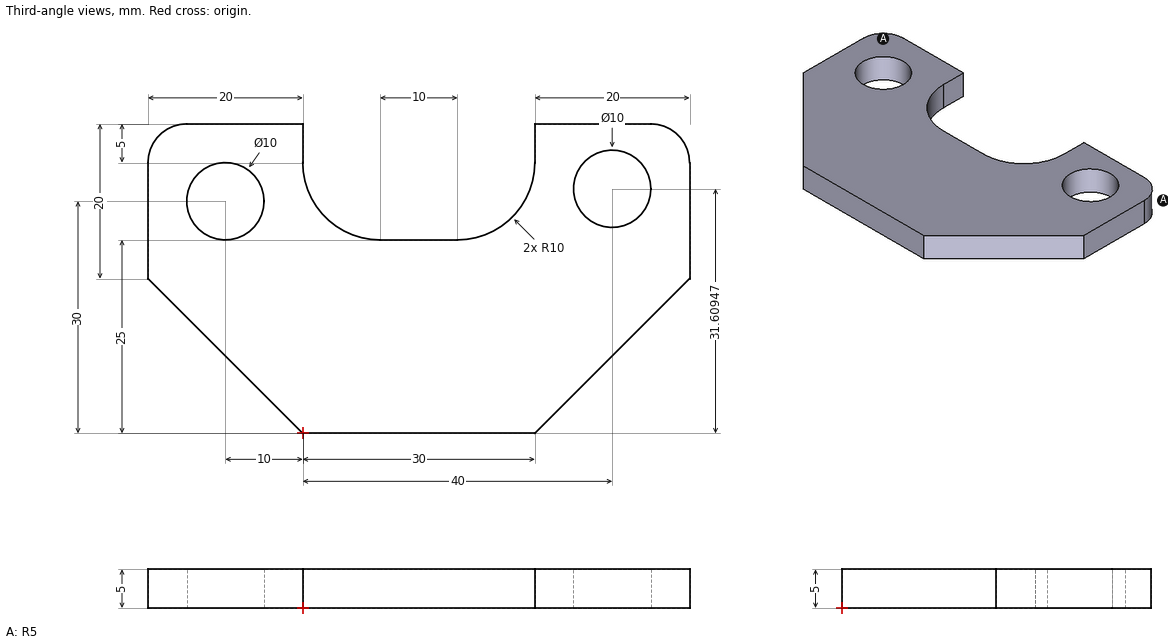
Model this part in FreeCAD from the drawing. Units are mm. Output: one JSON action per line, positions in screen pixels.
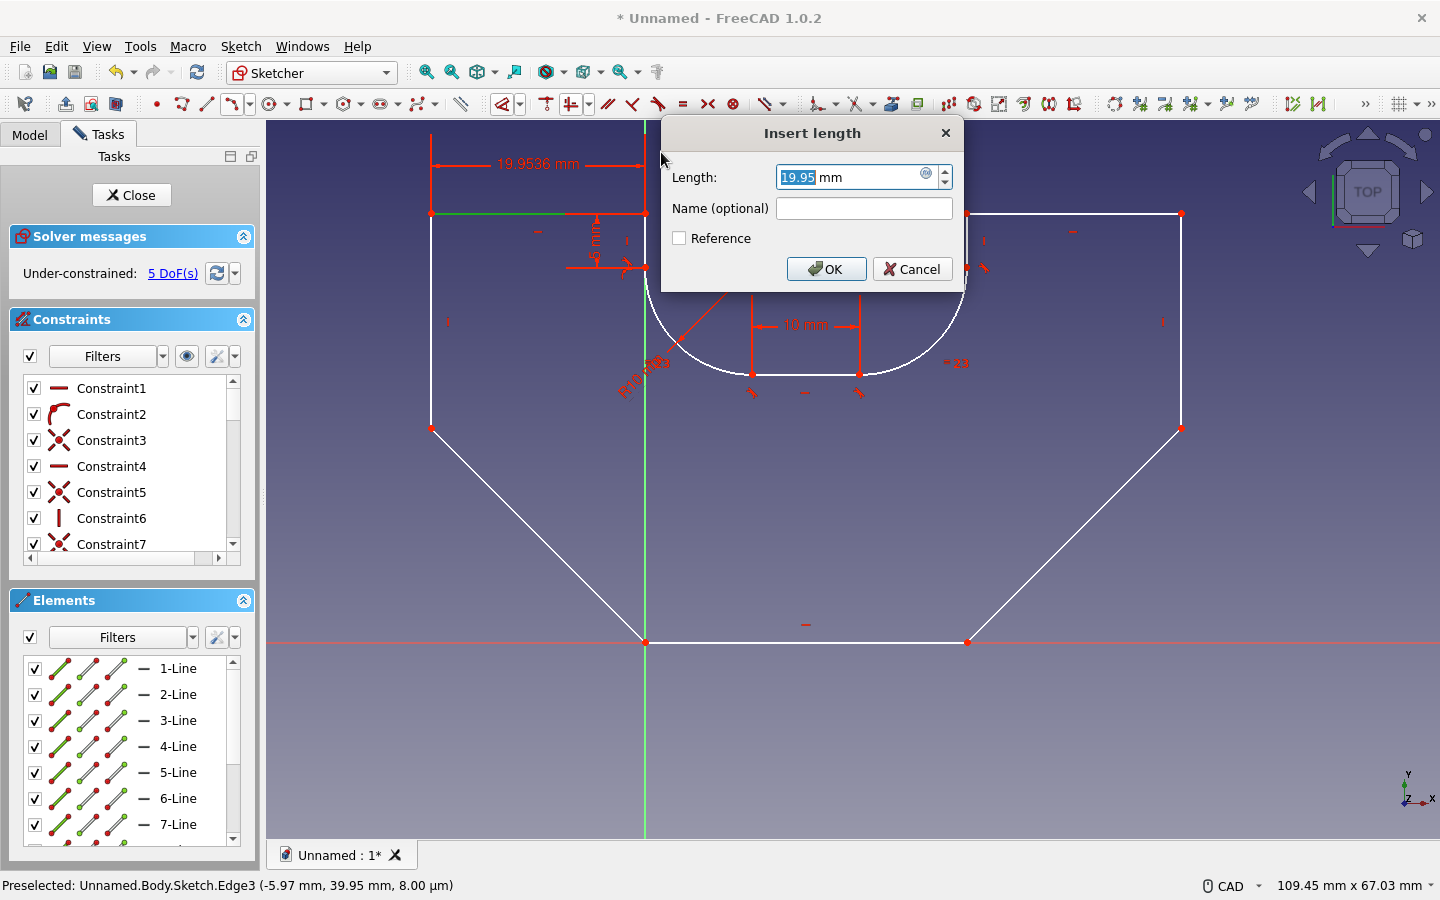
{"action": "type", "text": "20"}
{"action": "key", "text": "Return"}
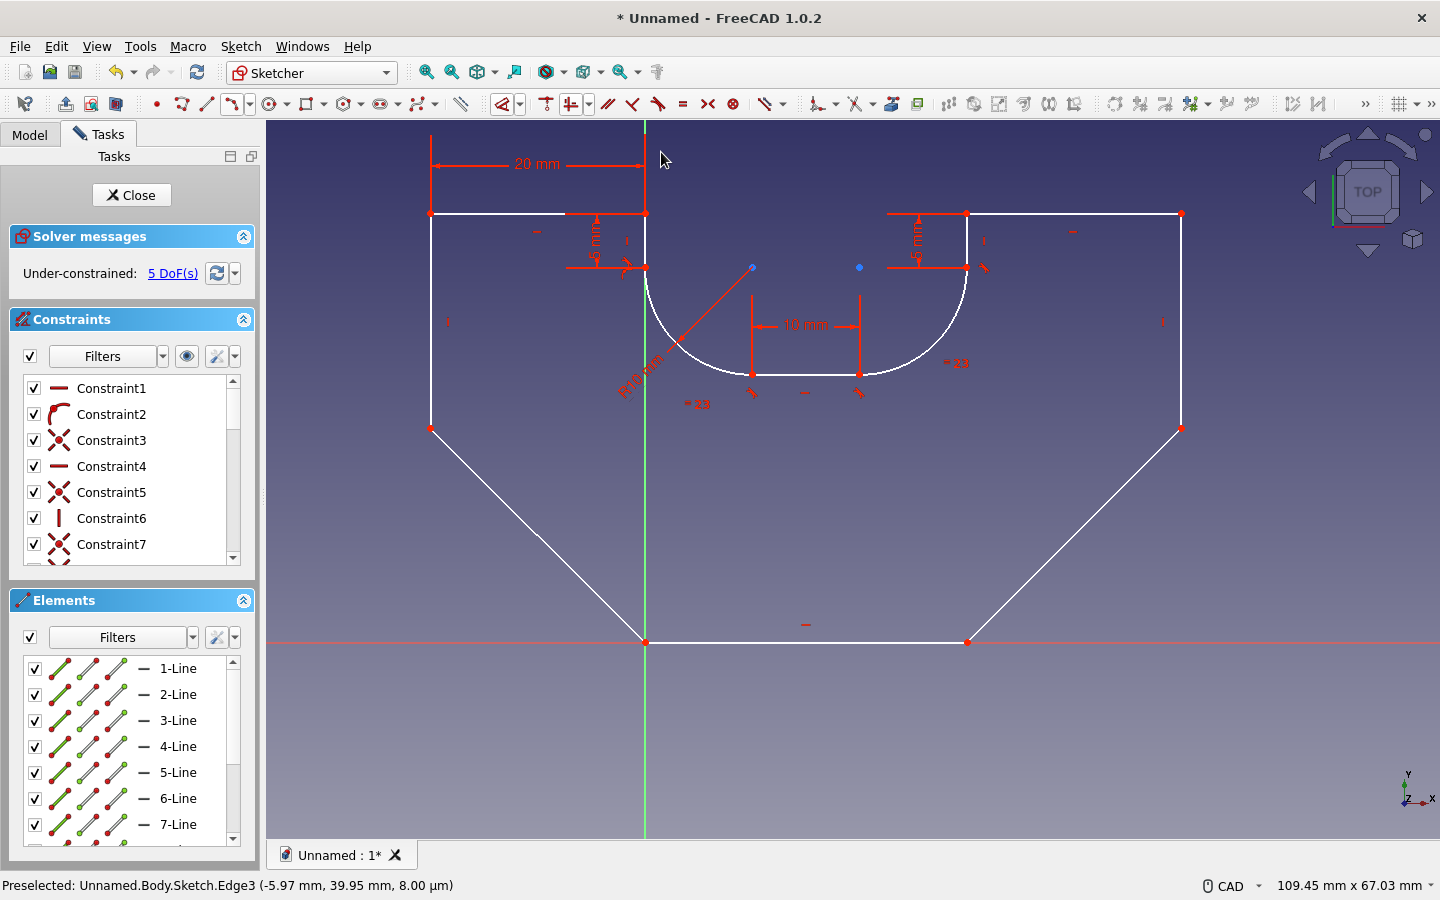
{"action": "left_click", "coordinate": [431, 278]}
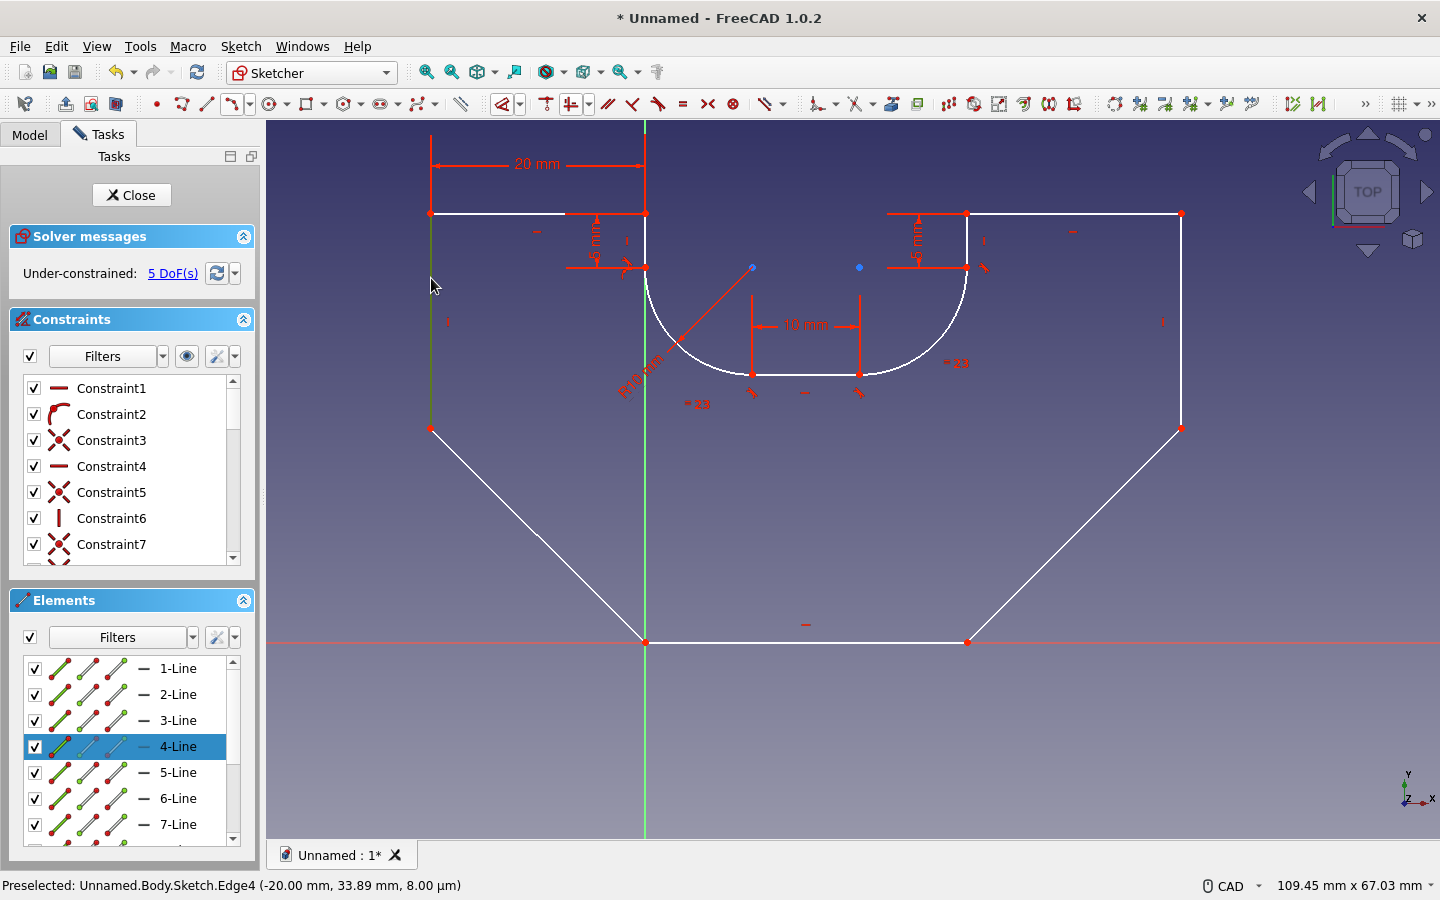
{"action": "key", "text": "i"}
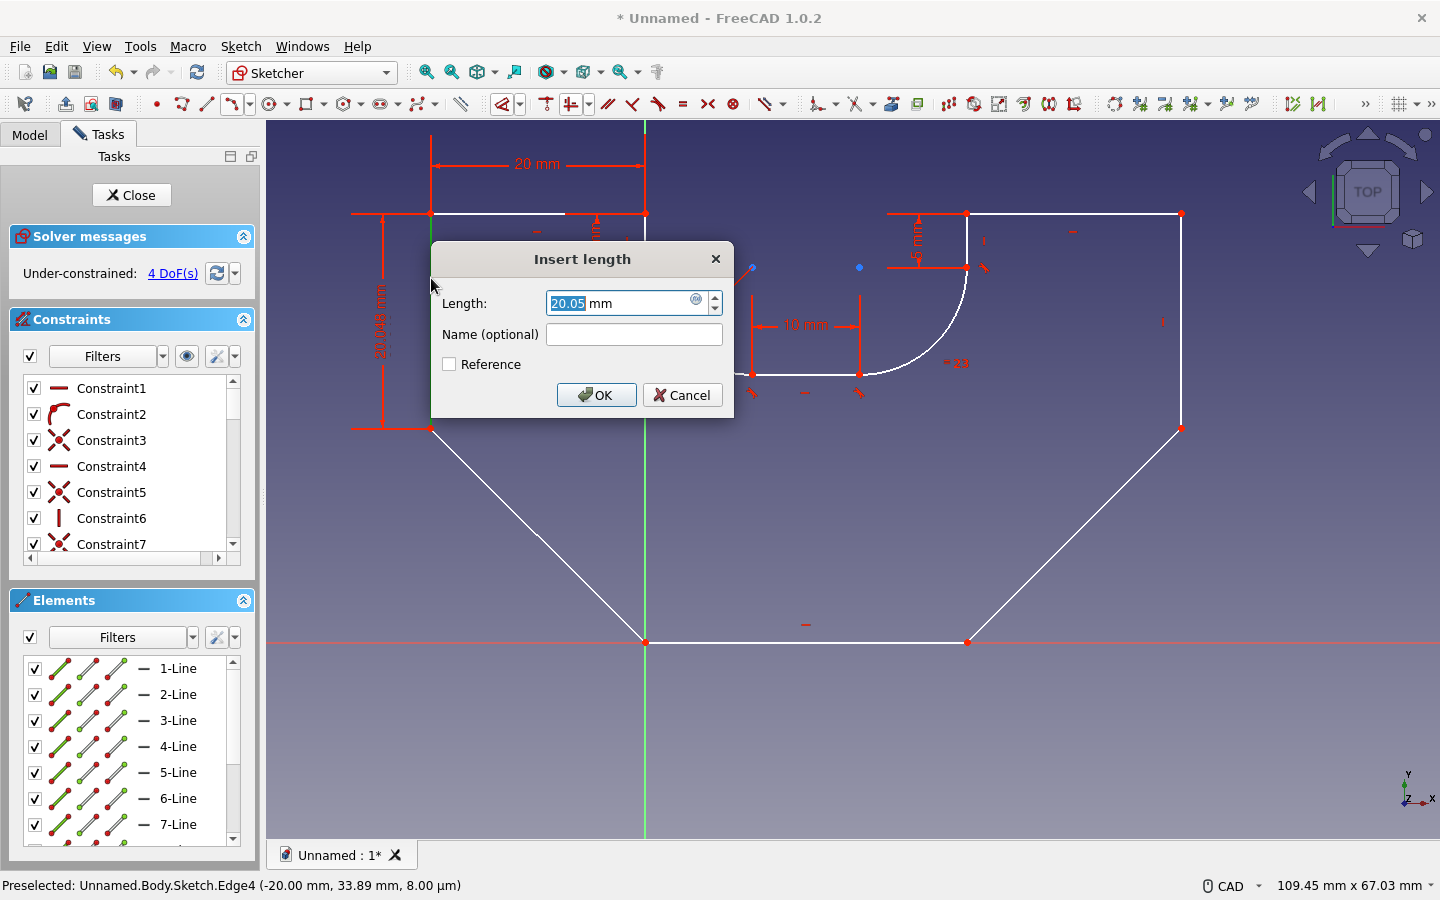
{"action": "type", "text": "20"}
{"action": "key", "text": "Return"}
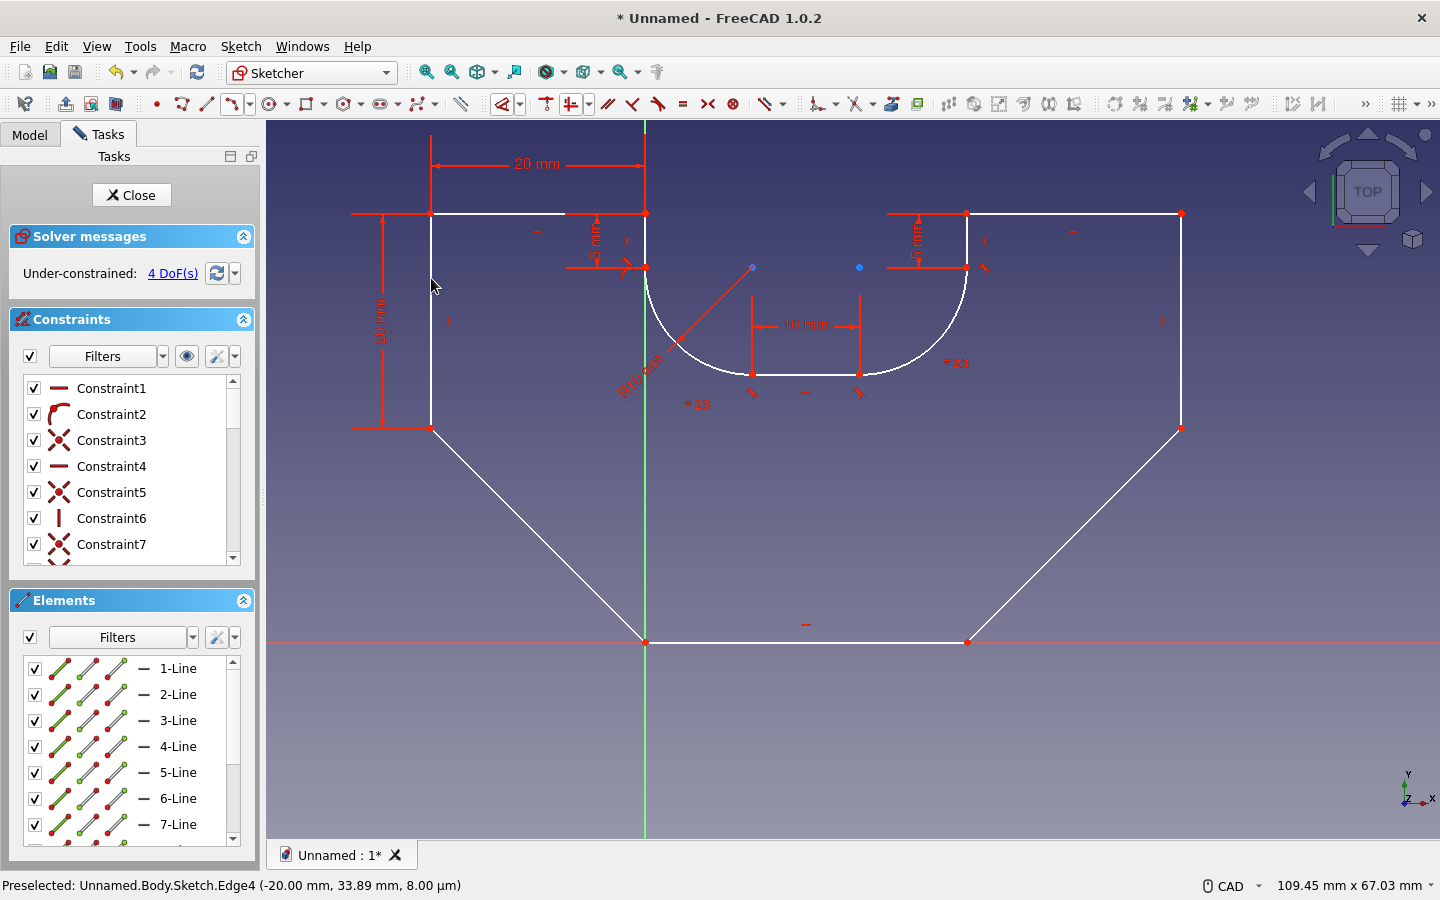
{"action": "left_click", "coordinate": [742, 643]}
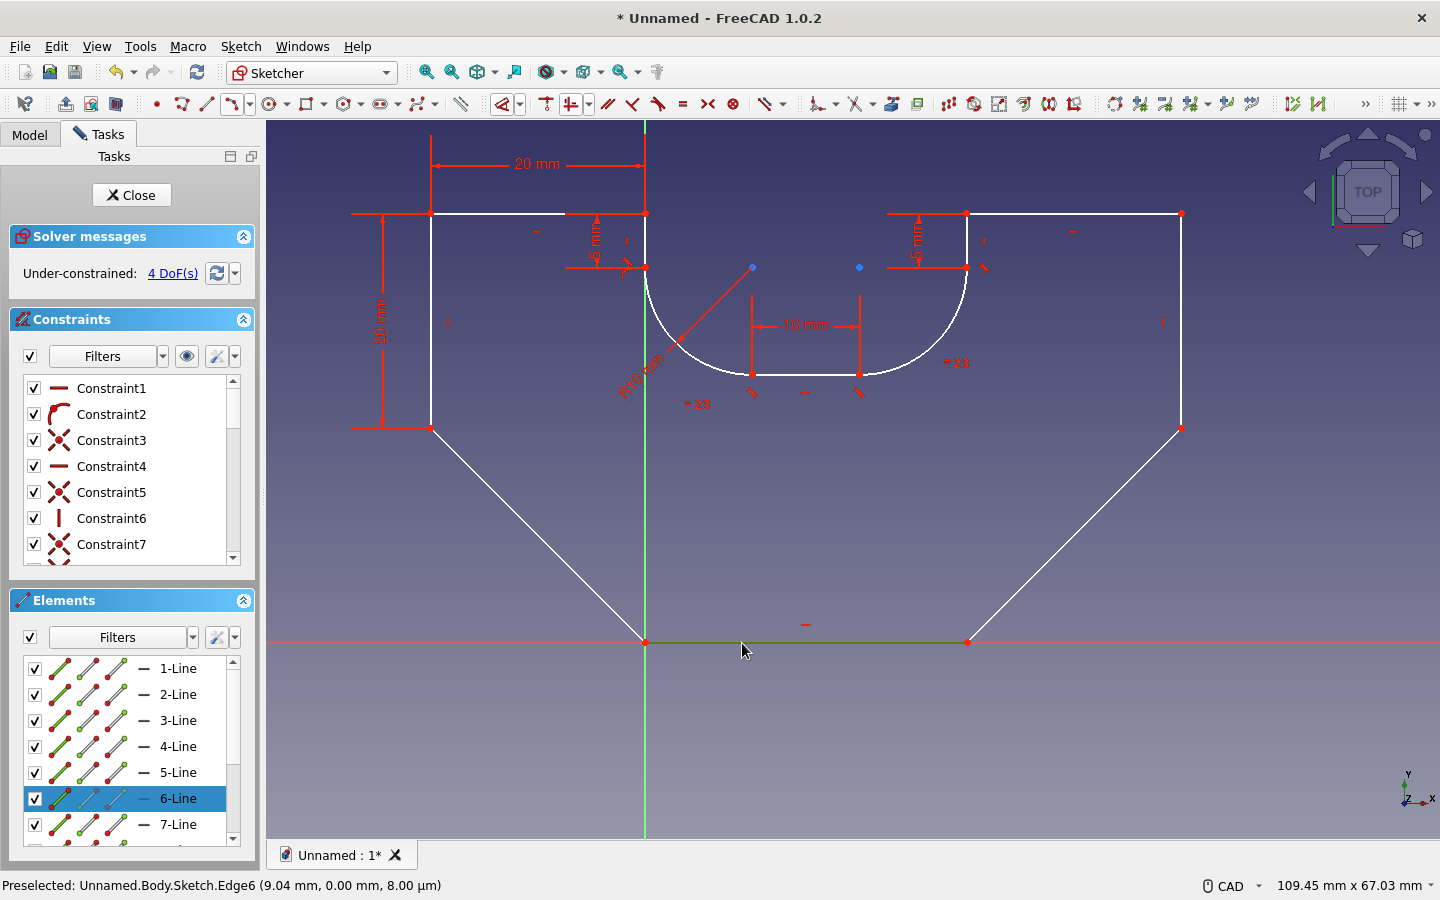
{"action": "left_click", "coordinate": [520, 104]}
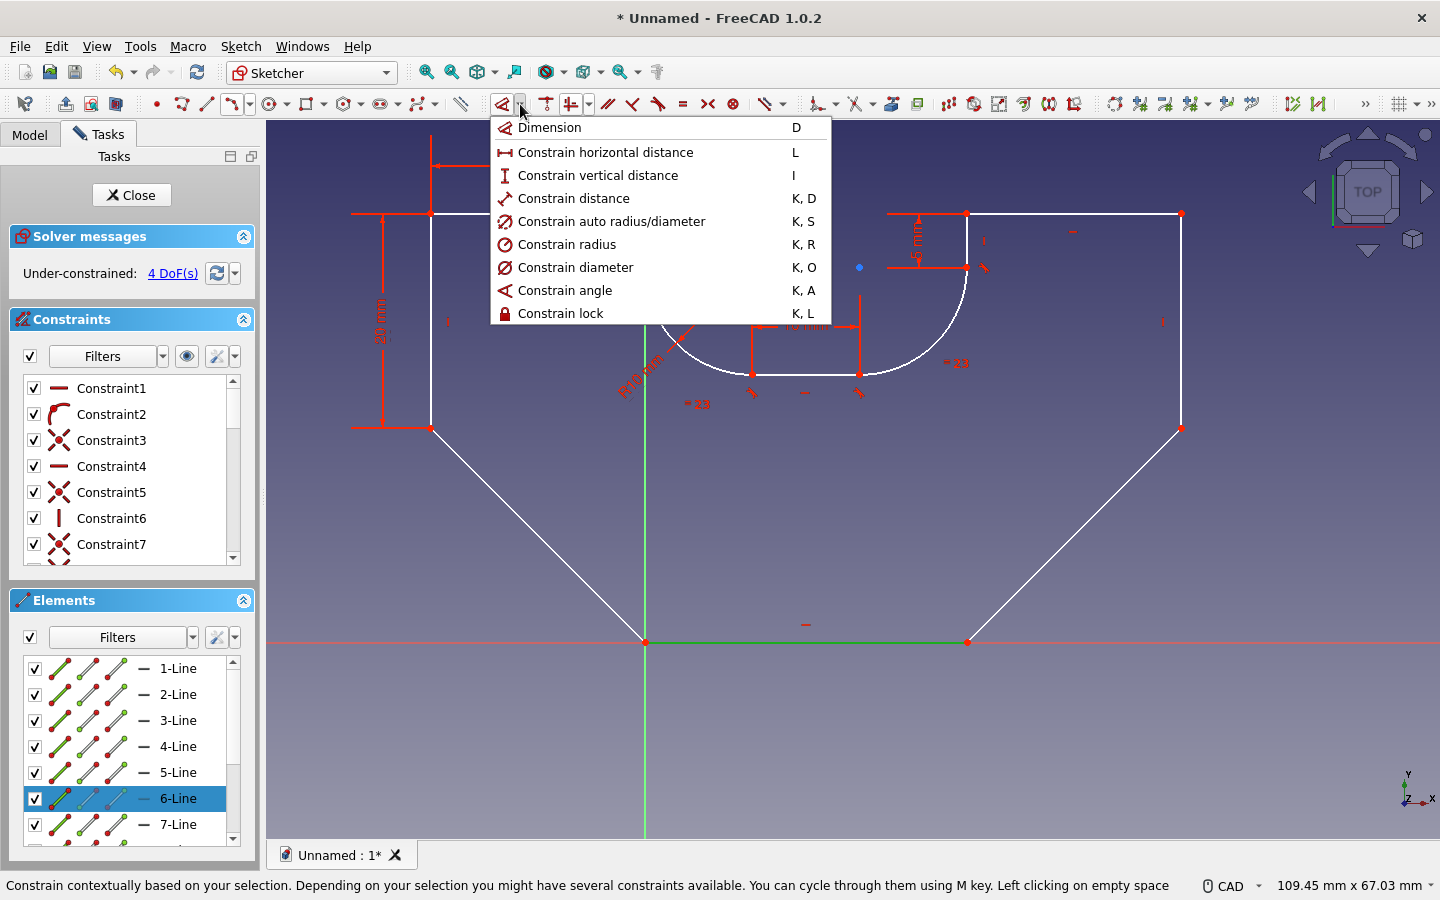
{"action": "left_click", "coordinate": [661, 152]}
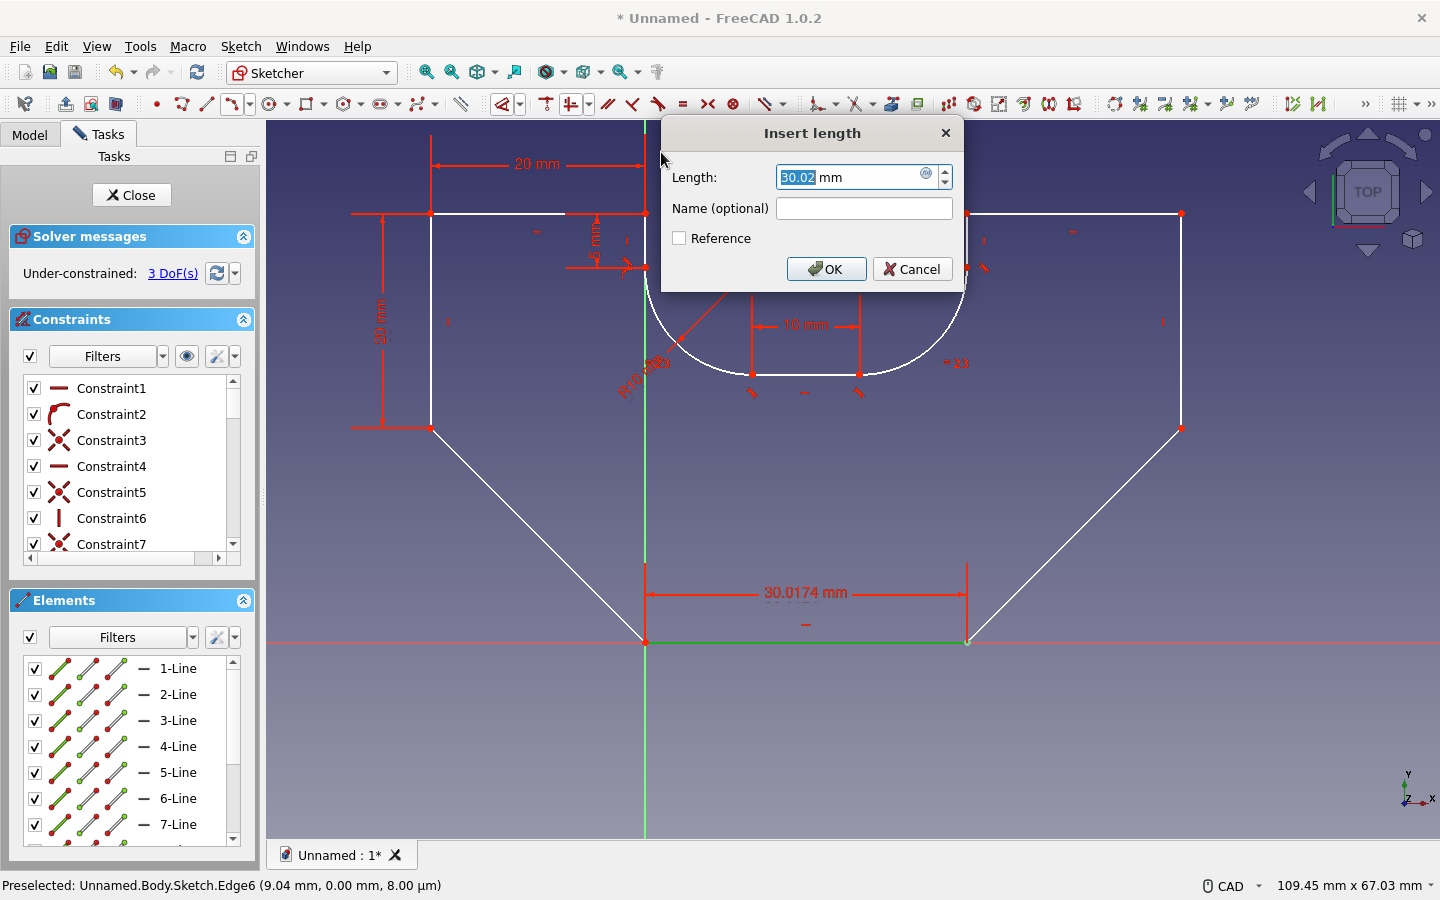
{"action": "type", "text": "30"}
{"action": "key", "text": "Return"}